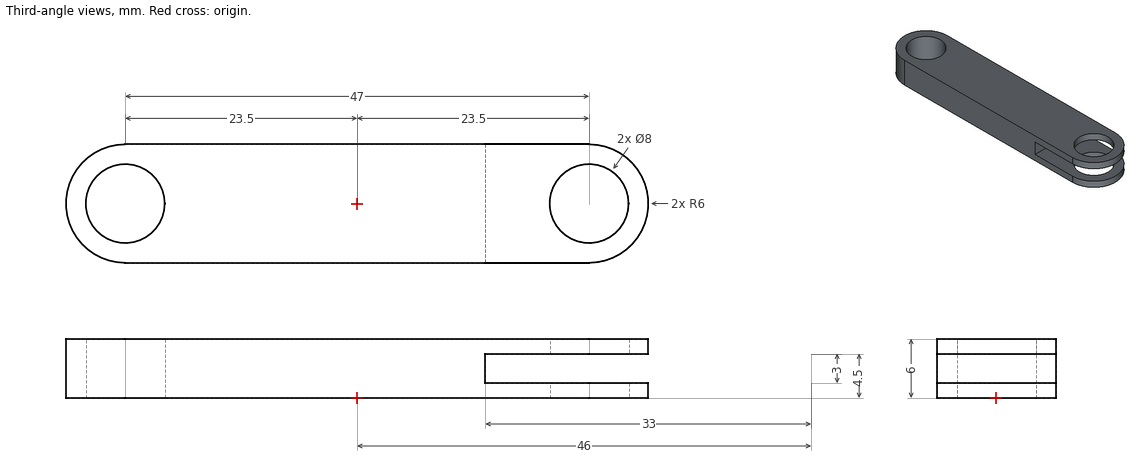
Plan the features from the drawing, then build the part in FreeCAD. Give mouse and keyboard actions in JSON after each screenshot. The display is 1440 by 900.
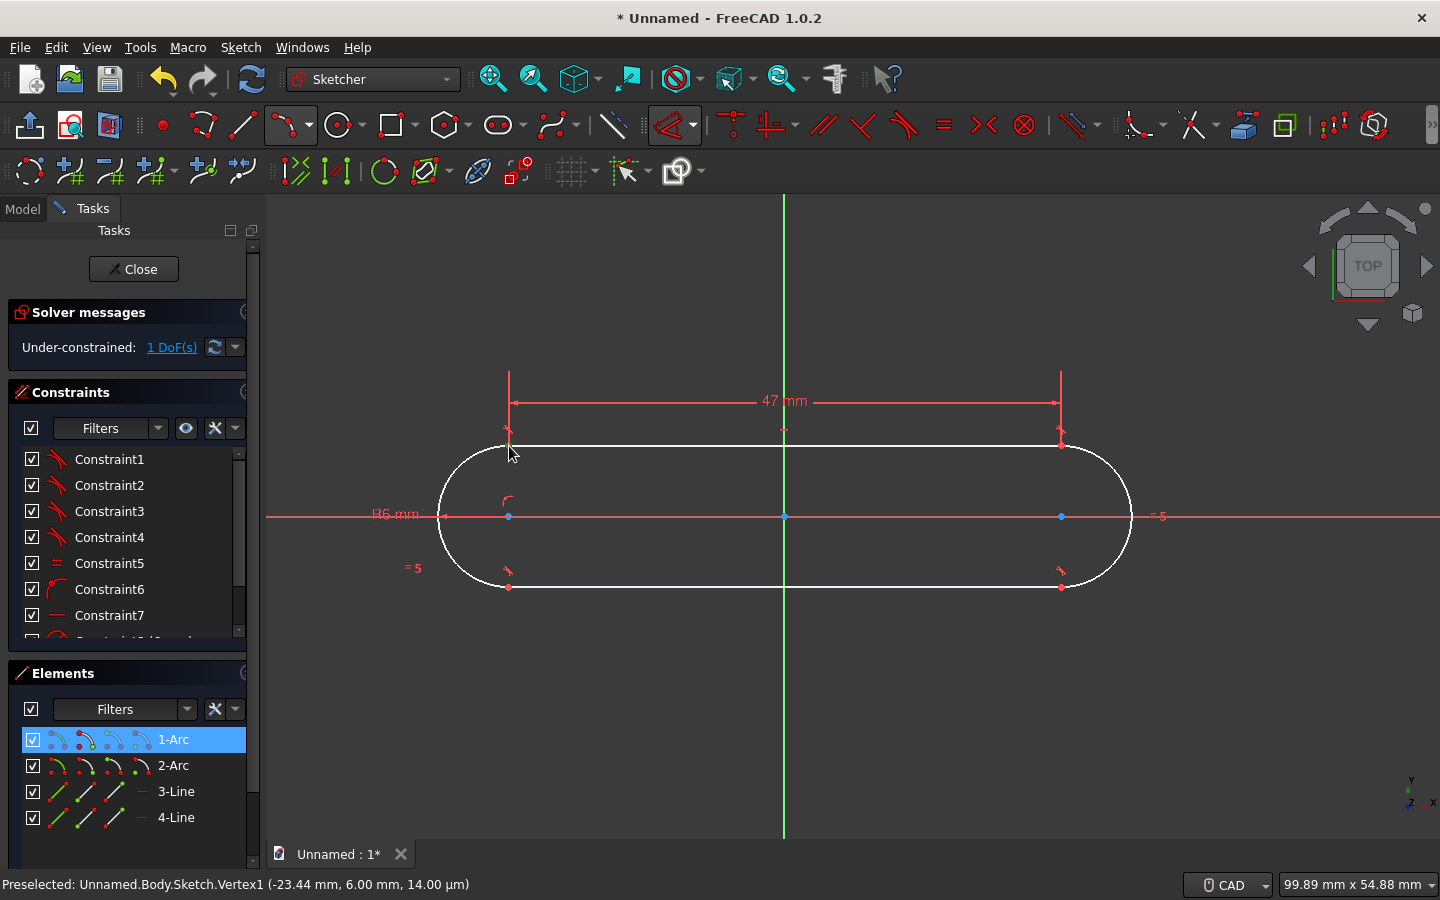
{"action": "key", "text": "l"}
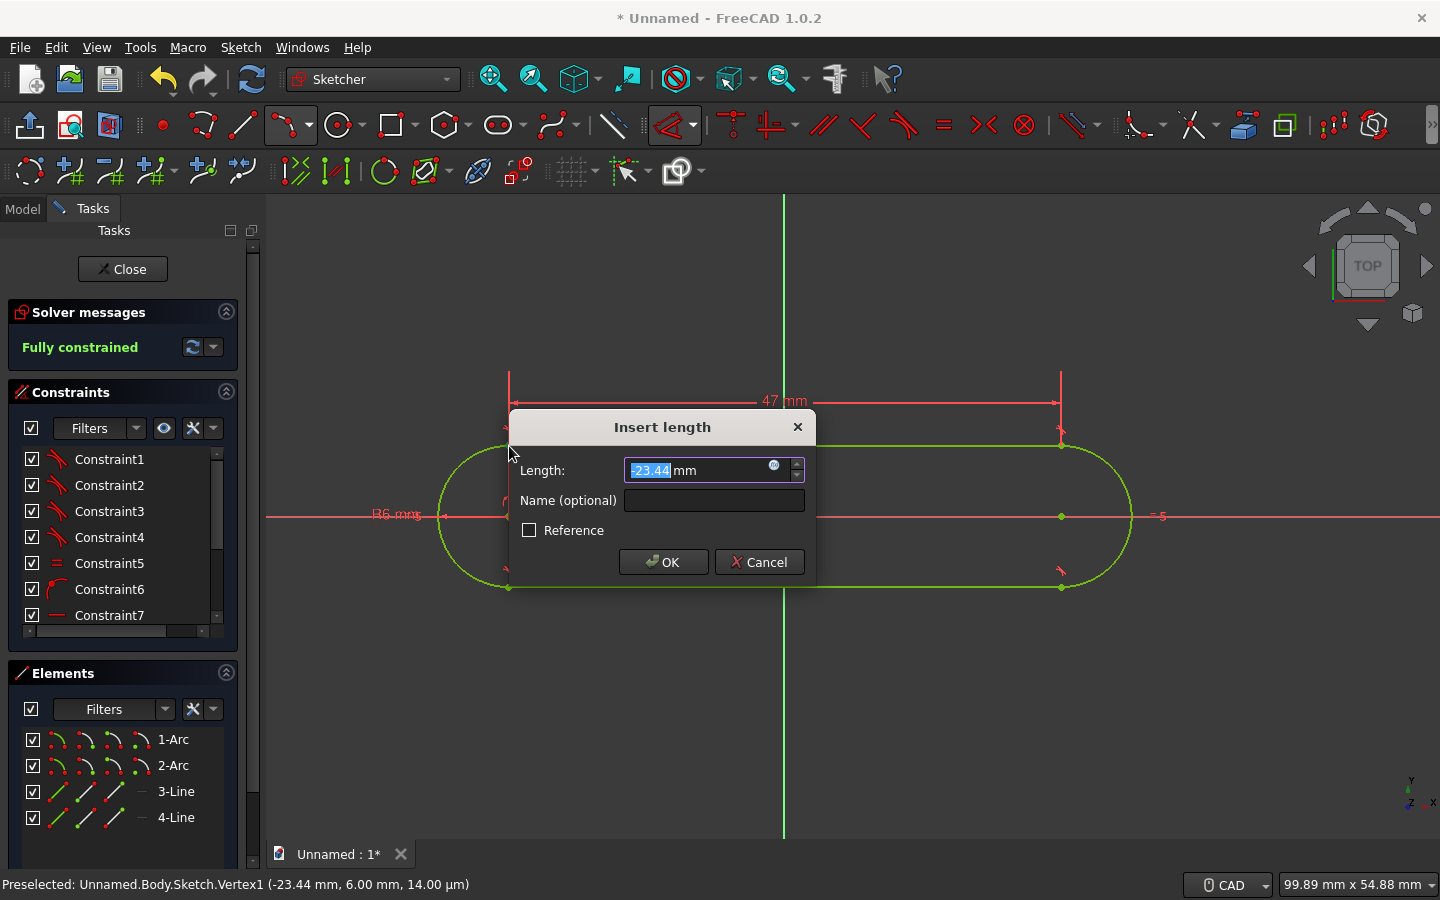
{"action": "type", "text": "-23.5"}
{"action": "key", "text": "Return"}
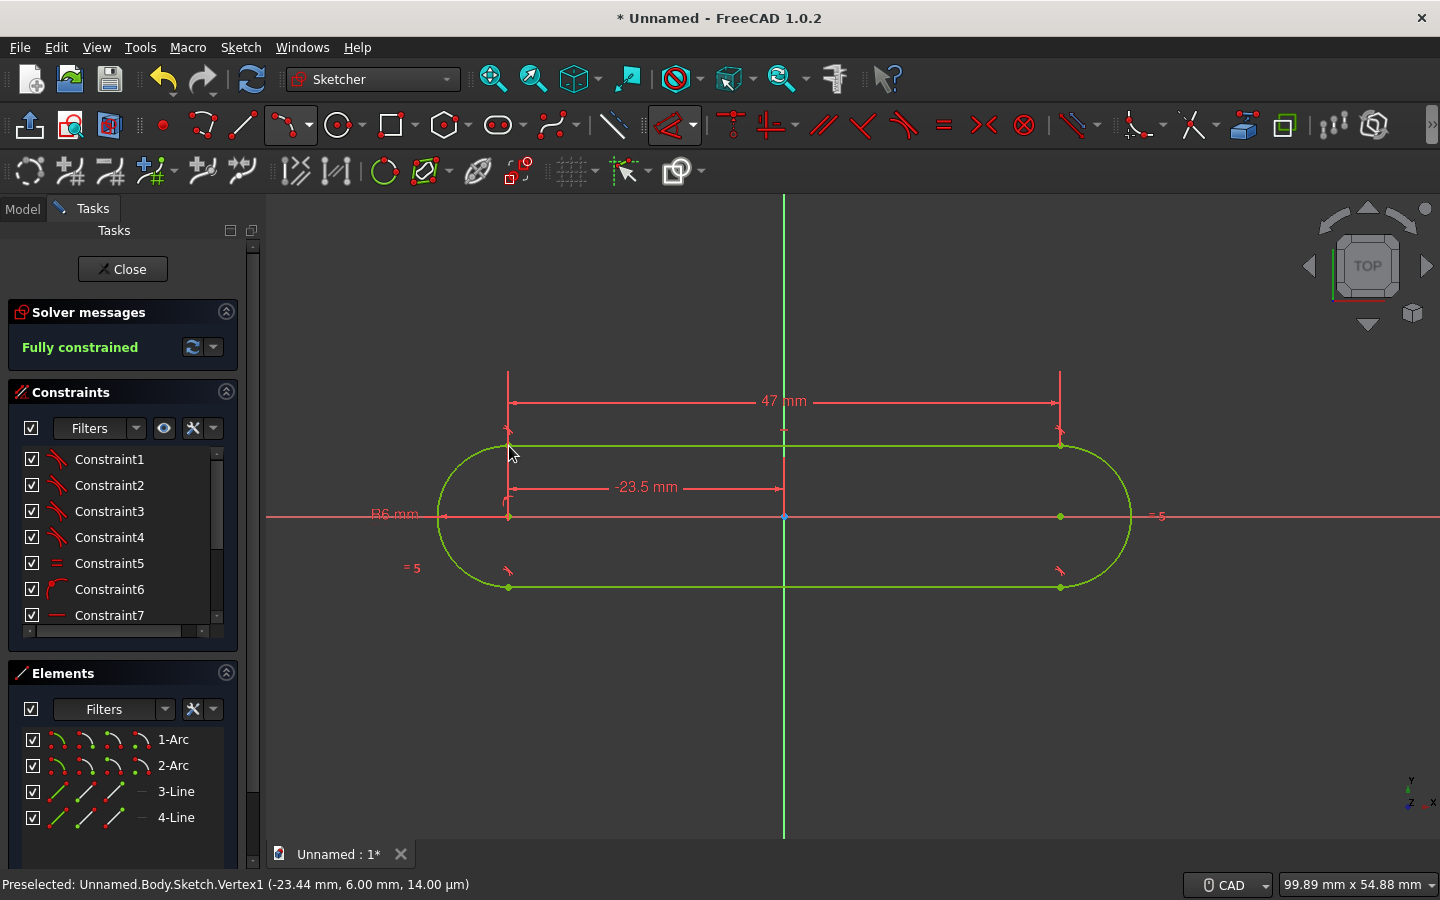
{"action": "left_click", "coordinate": [123, 269]}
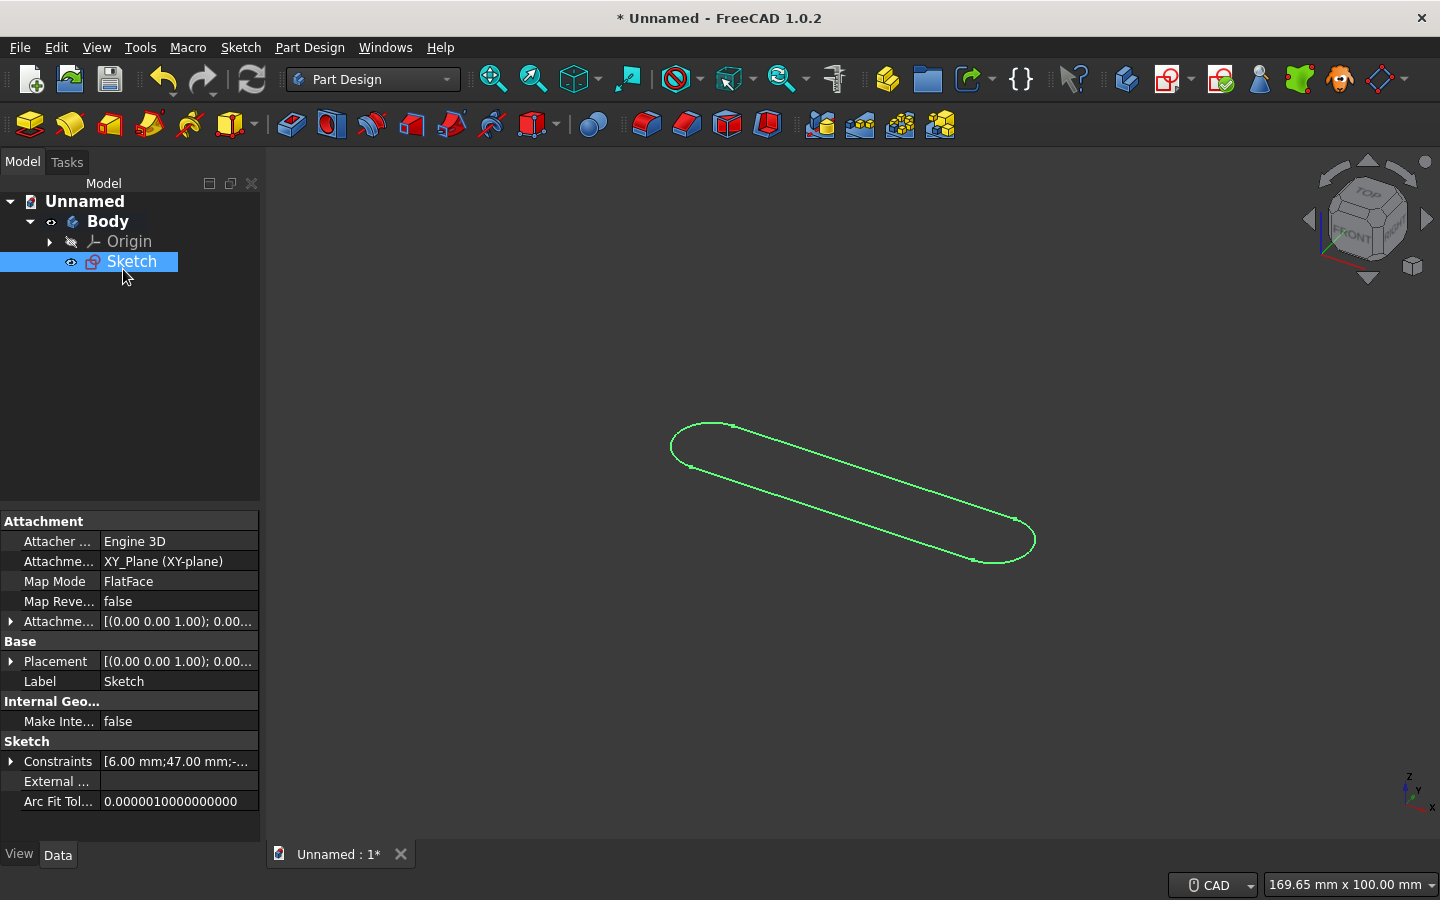
{"action": "left_click", "coordinate": [30, 124]}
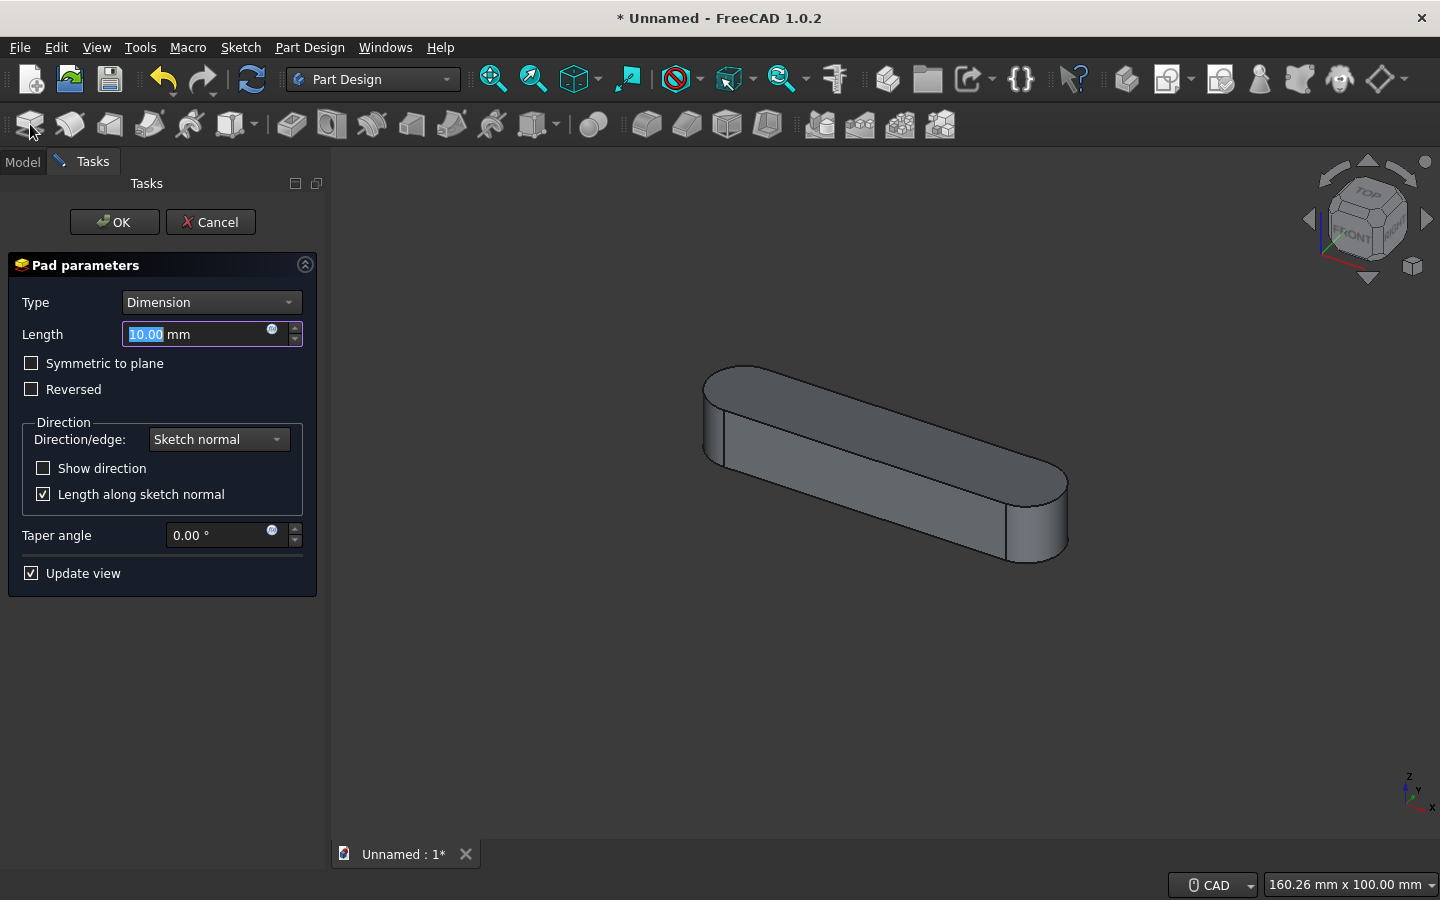
{"action": "type", "text": "6"}
{"action": "key", "text": "Tab"}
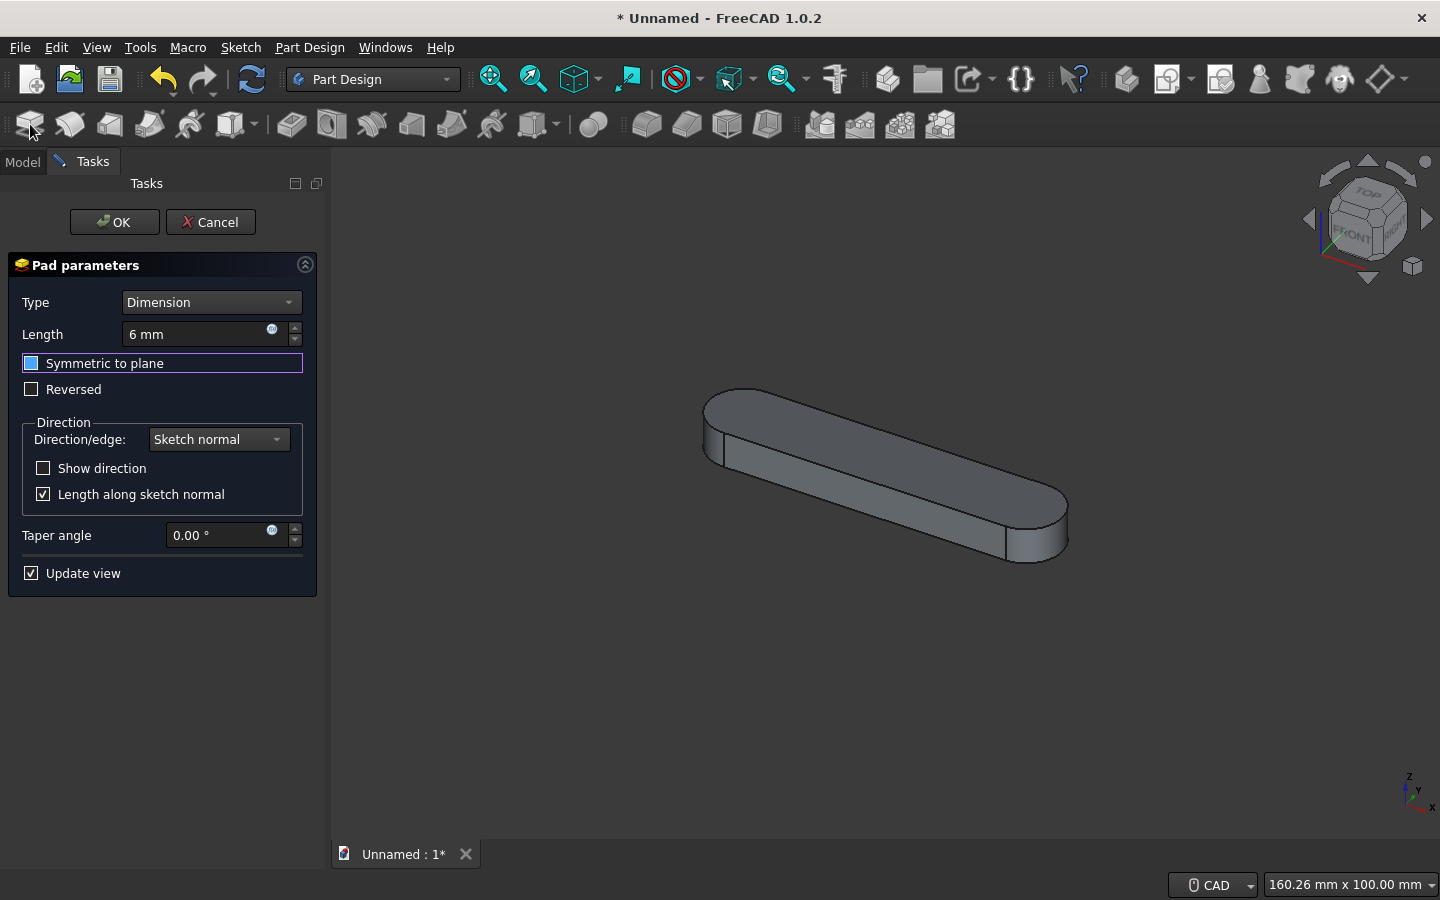
{"action": "left_click", "coordinate": [115, 222]}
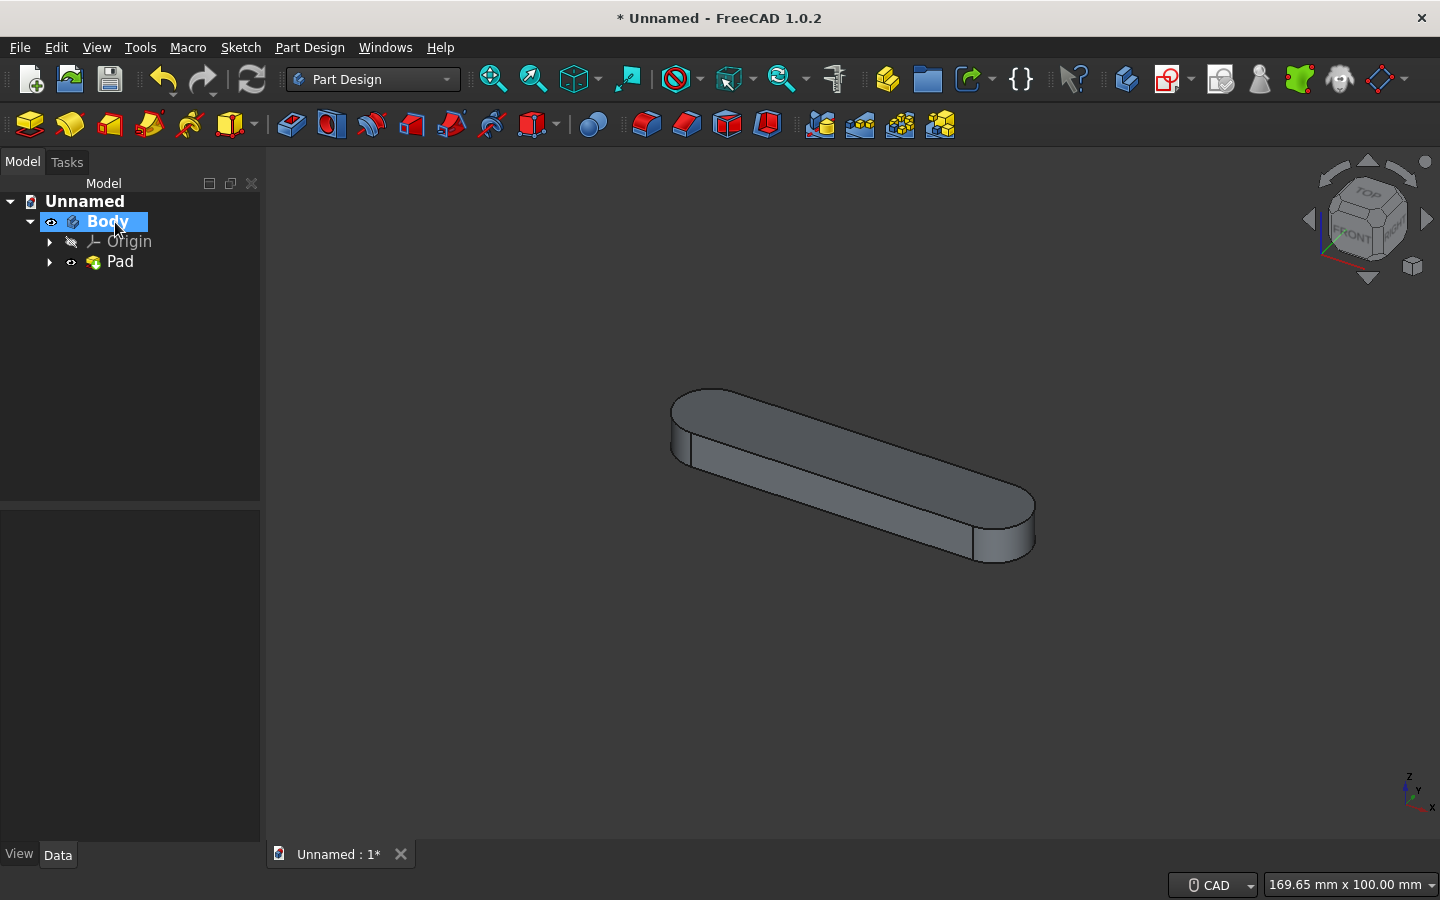
{"action": "left_click", "coordinate": [494, 80]}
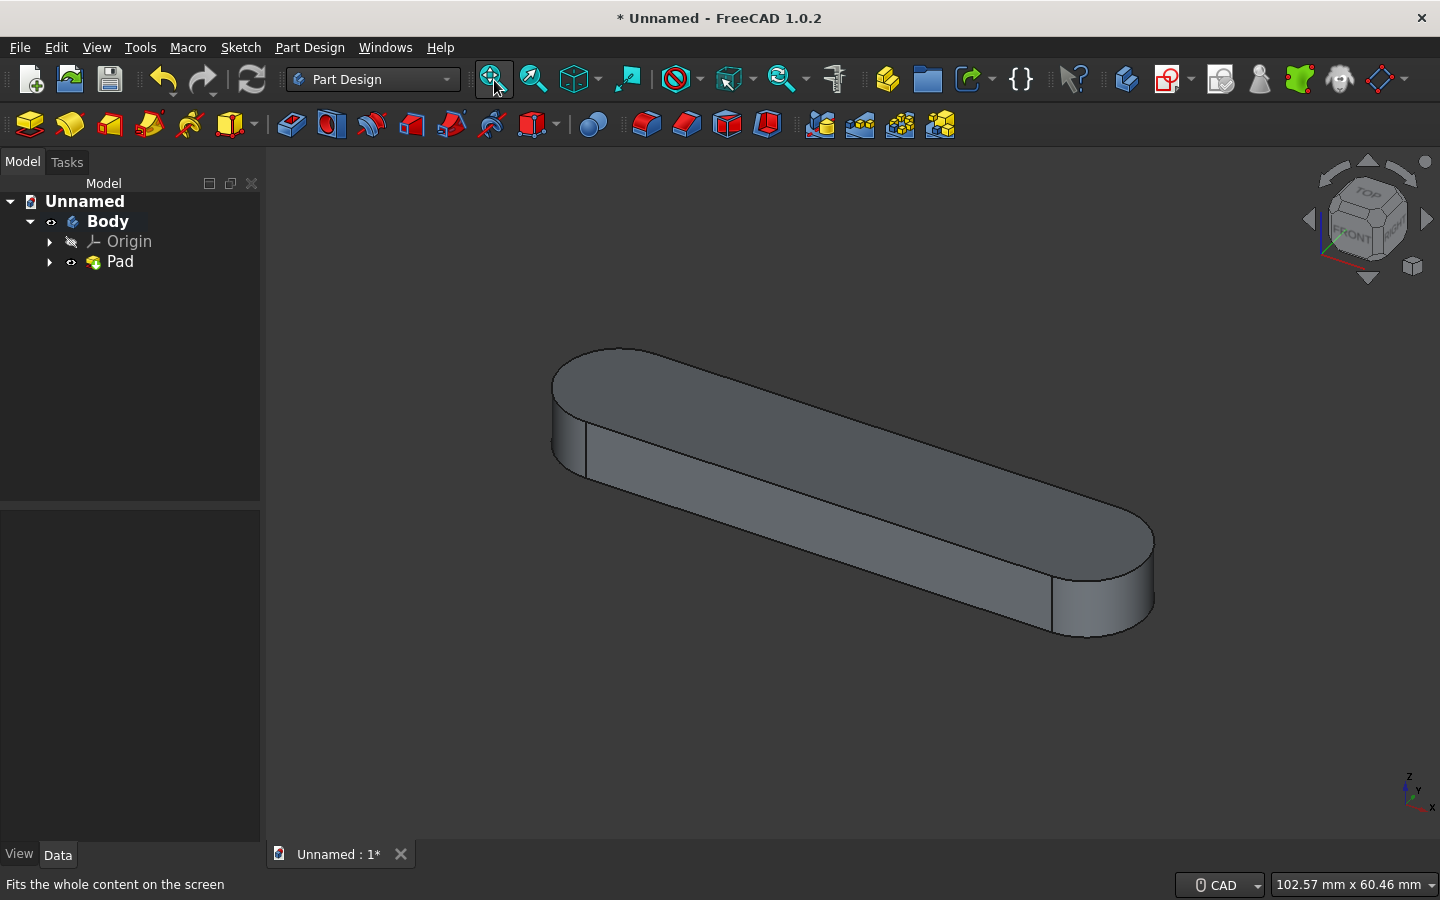
{"action": "key", "text": "4"}